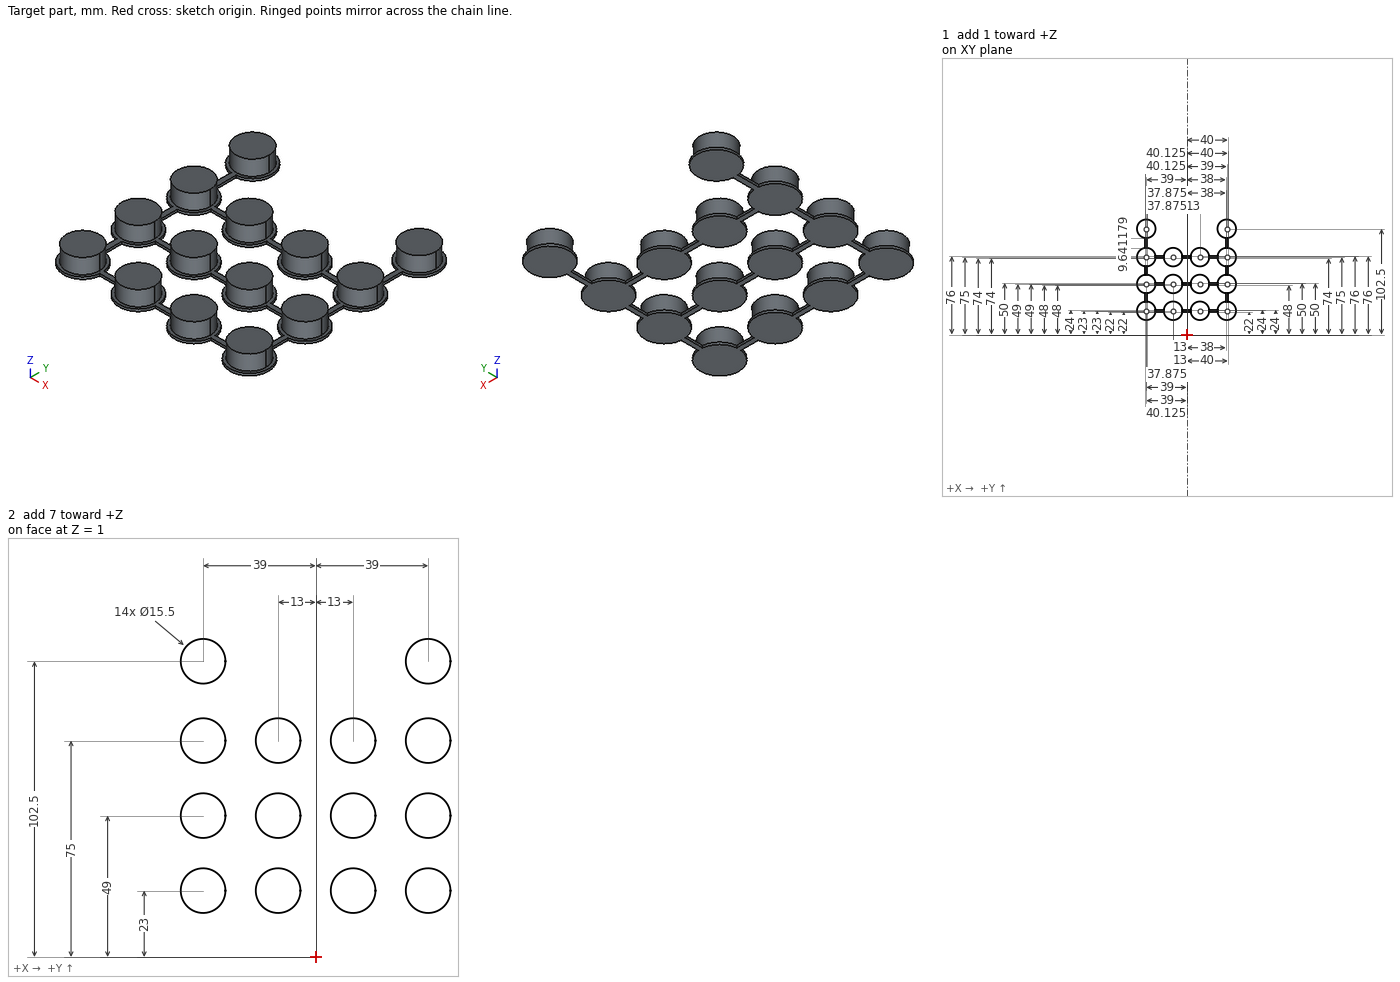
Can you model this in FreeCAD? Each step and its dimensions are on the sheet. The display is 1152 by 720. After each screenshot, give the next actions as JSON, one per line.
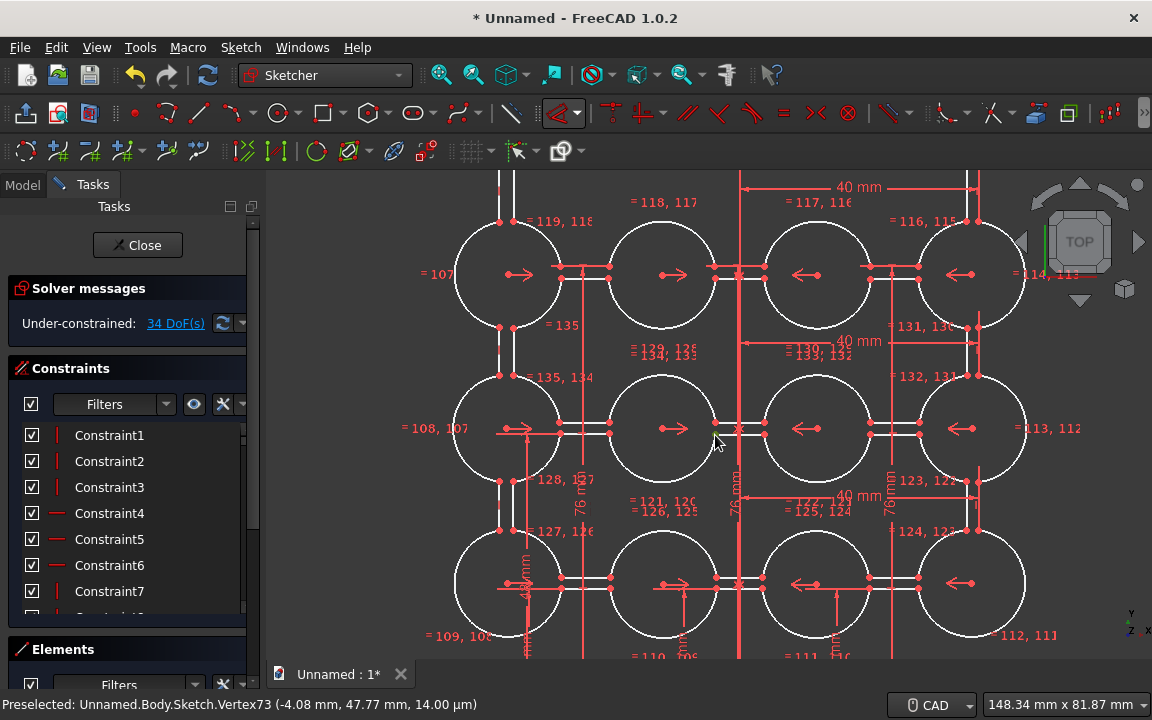
{"action": "left_click", "coordinate": [580, 114]}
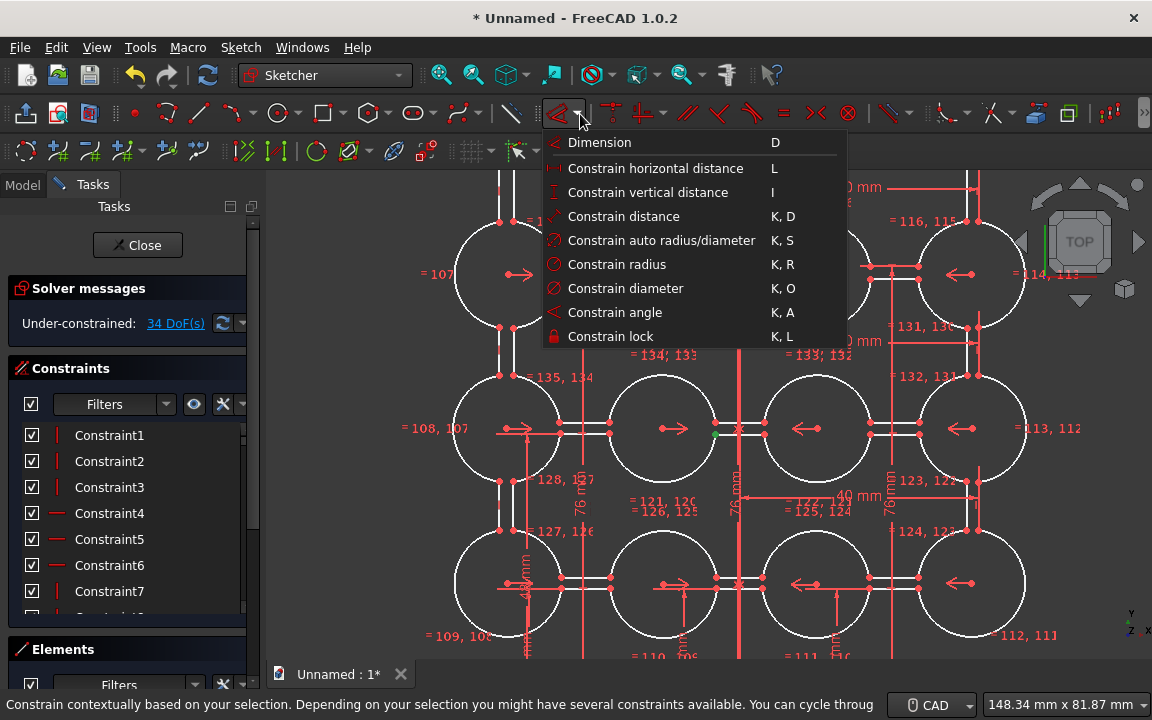
{"action": "left_click", "coordinate": [695, 192]}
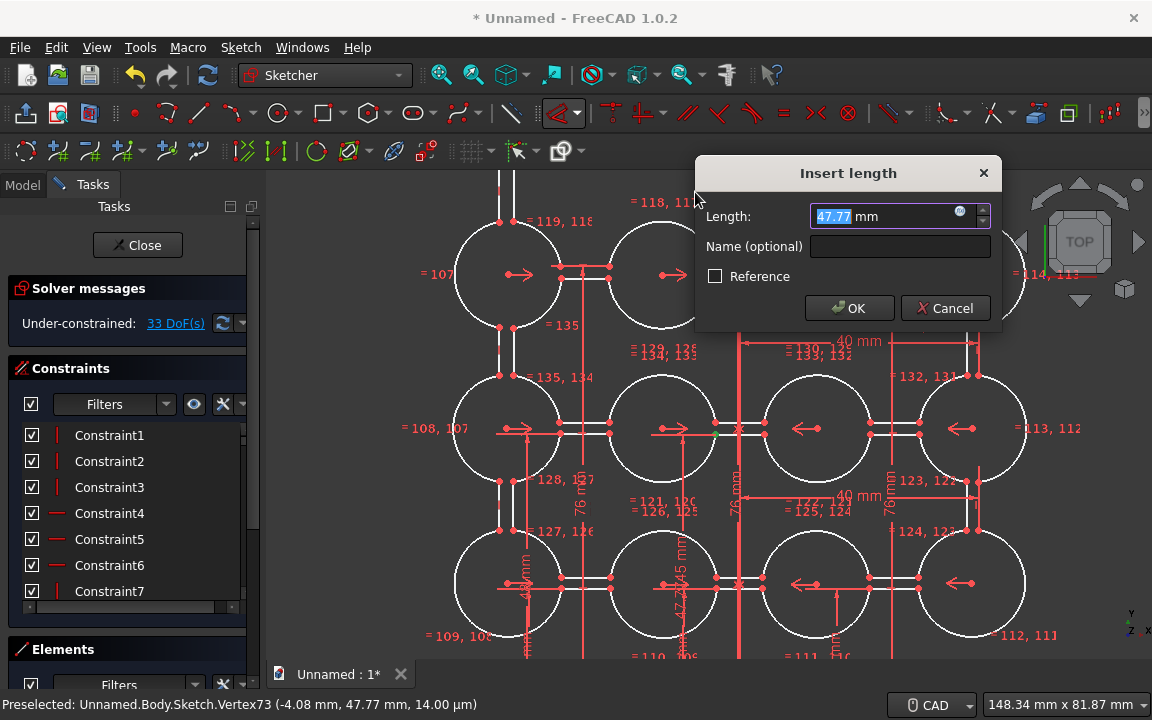
{"action": "type", "text": "48"}
{"action": "key", "text": "Return"}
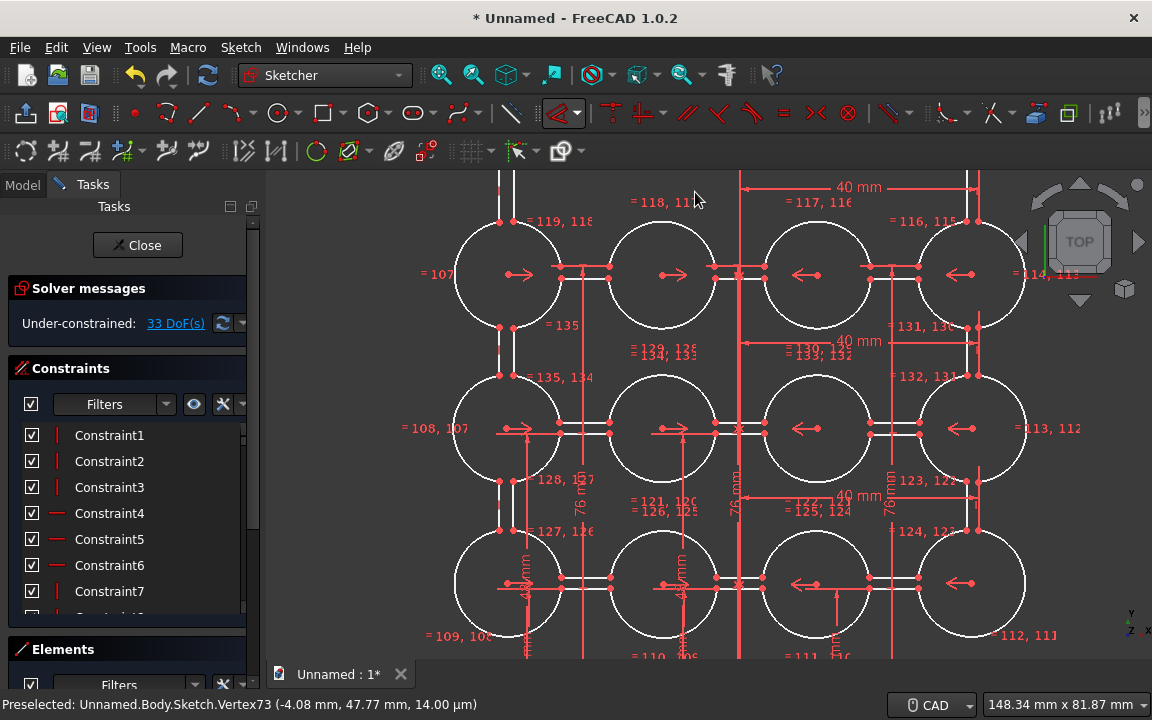
{"action": "left_click", "coordinate": [871, 435]}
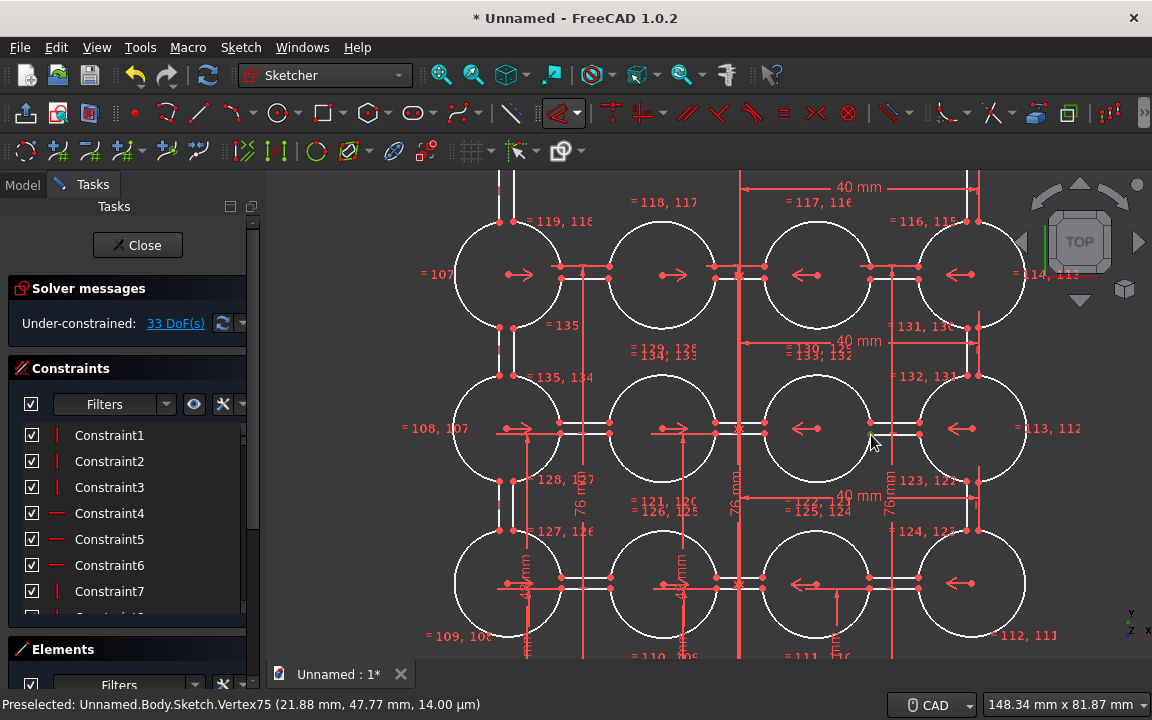
{"action": "left_click", "coordinate": [580, 114]}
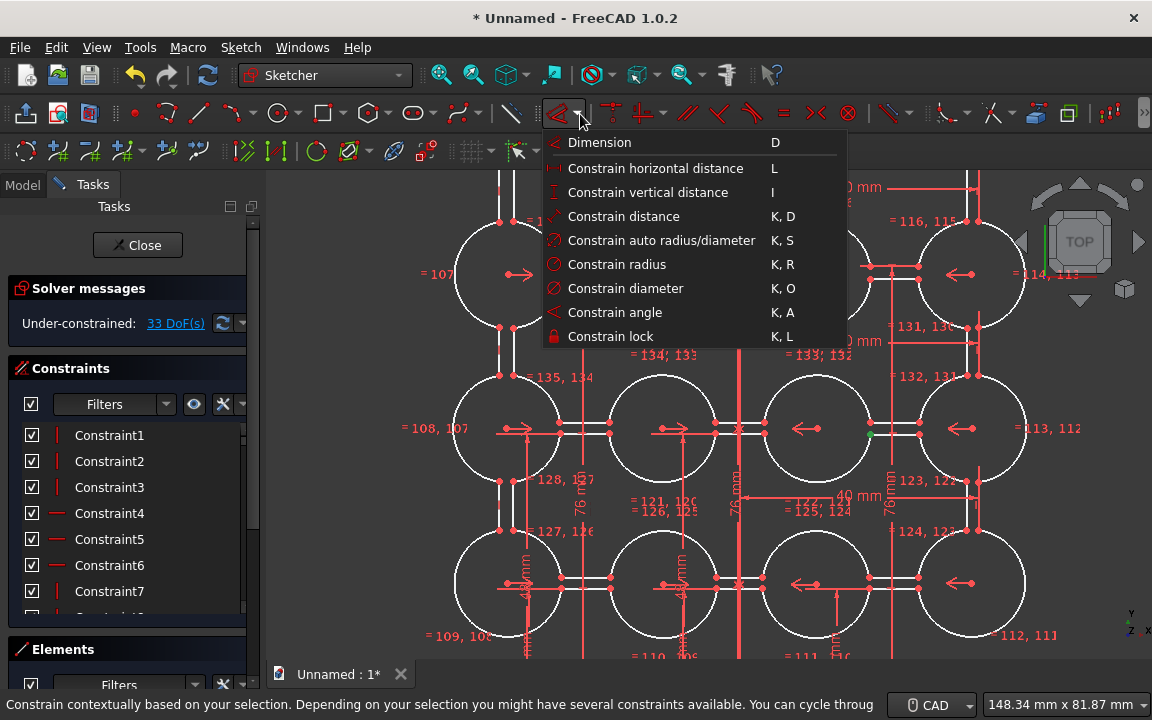
{"action": "left_click", "coordinate": [695, 192]}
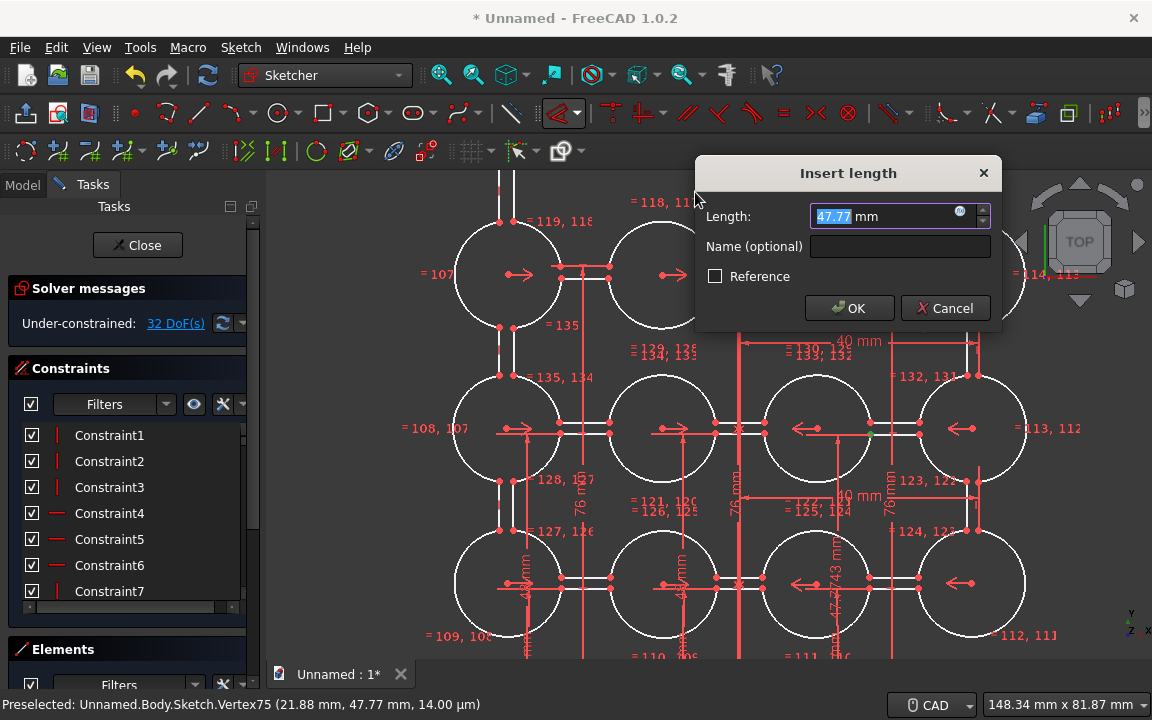
{"action": "type", "text": "48"}
{"action": "key", "text": "Return"}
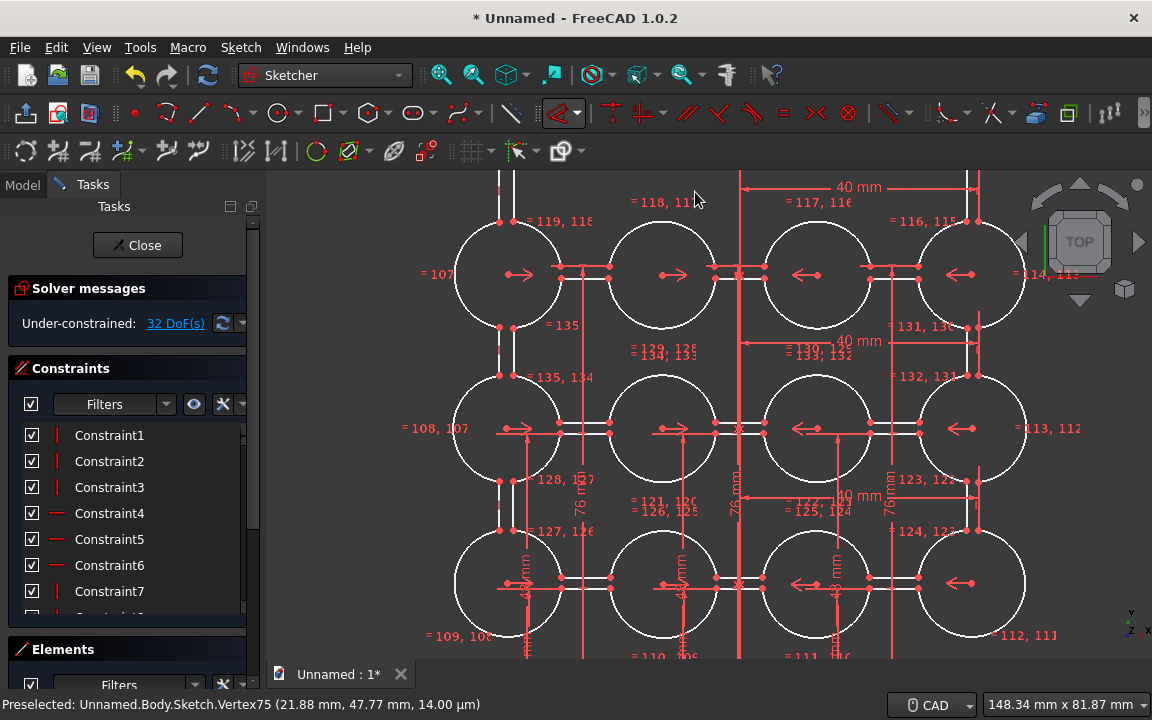
{"action": "left_click", "coordinate": [967, 482]}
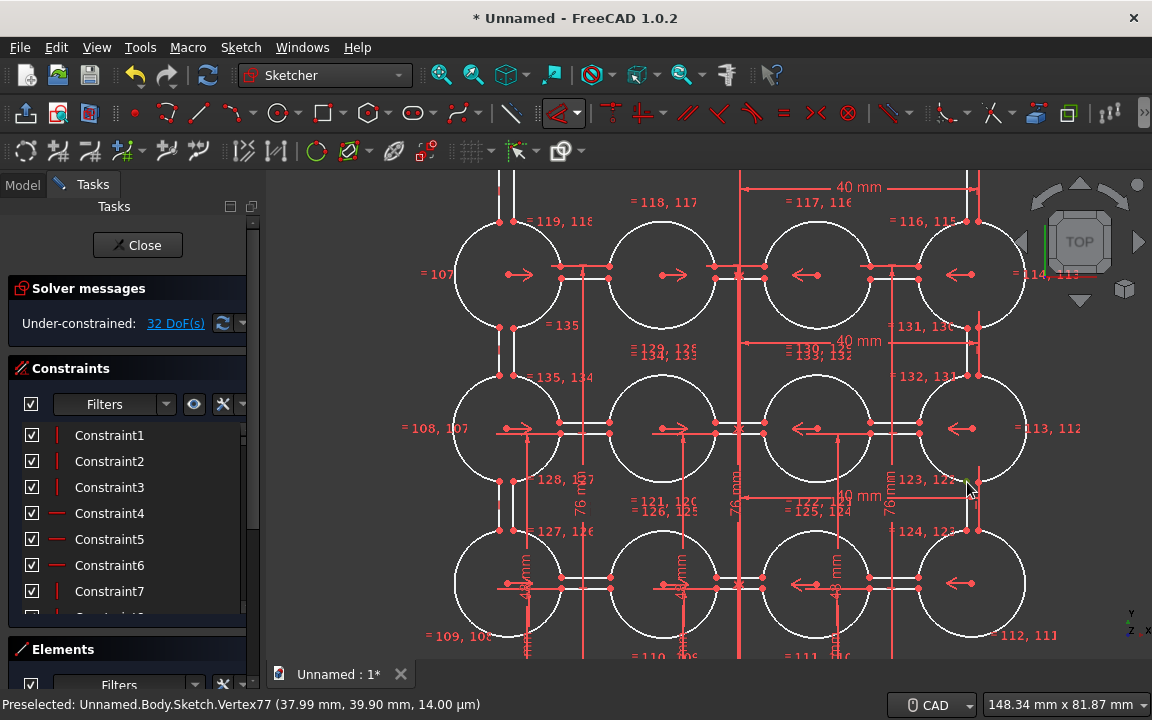
{"action": "left_click", "coordinate": [580, 114]}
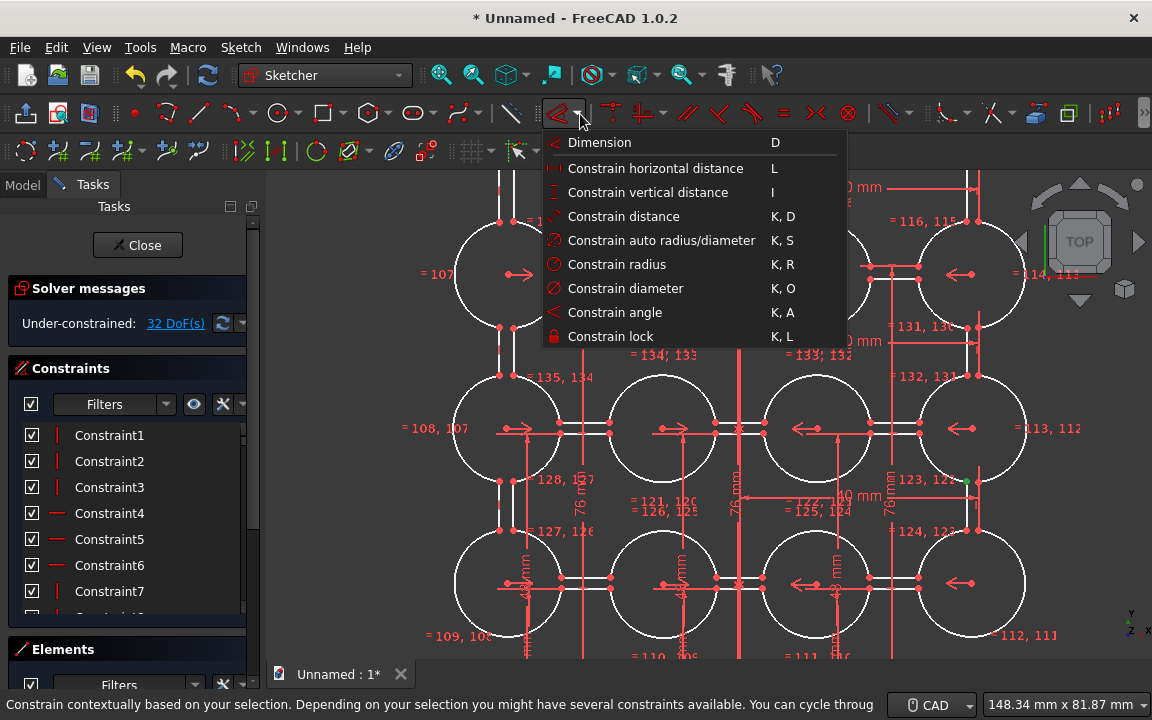
{"action": "left_click", "coordinate": [695, 168]}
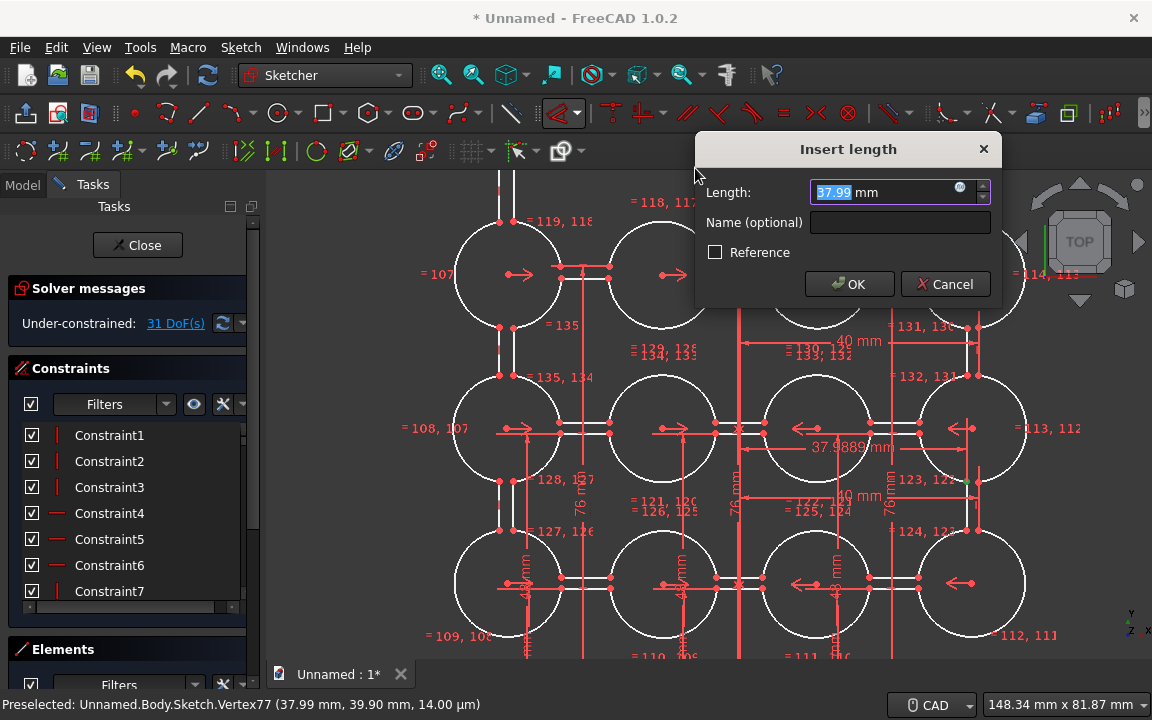
{"action": "type", "text": "38"}
{"action": "key", "text": "Return"}